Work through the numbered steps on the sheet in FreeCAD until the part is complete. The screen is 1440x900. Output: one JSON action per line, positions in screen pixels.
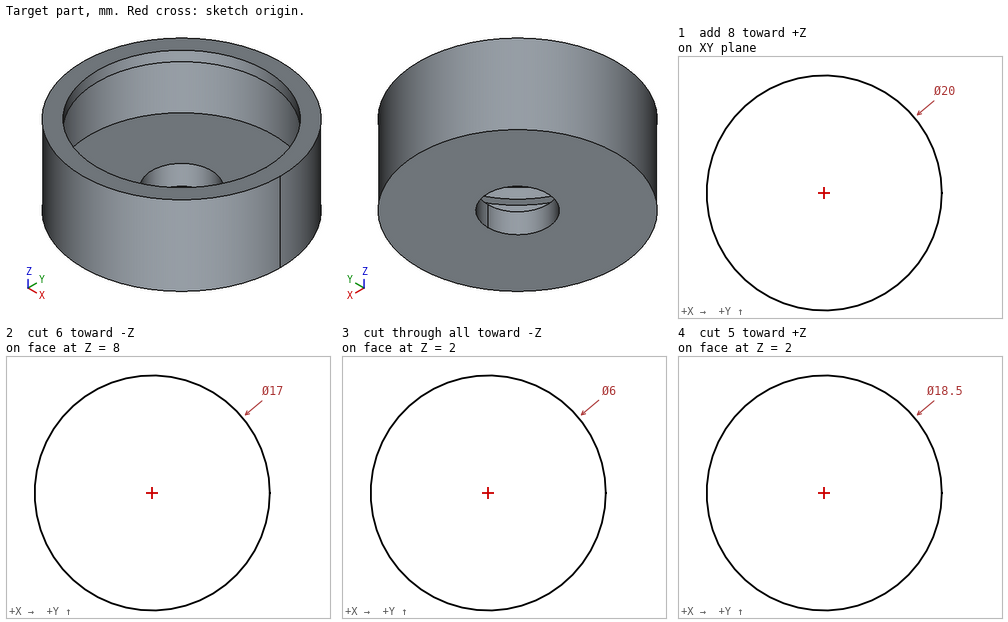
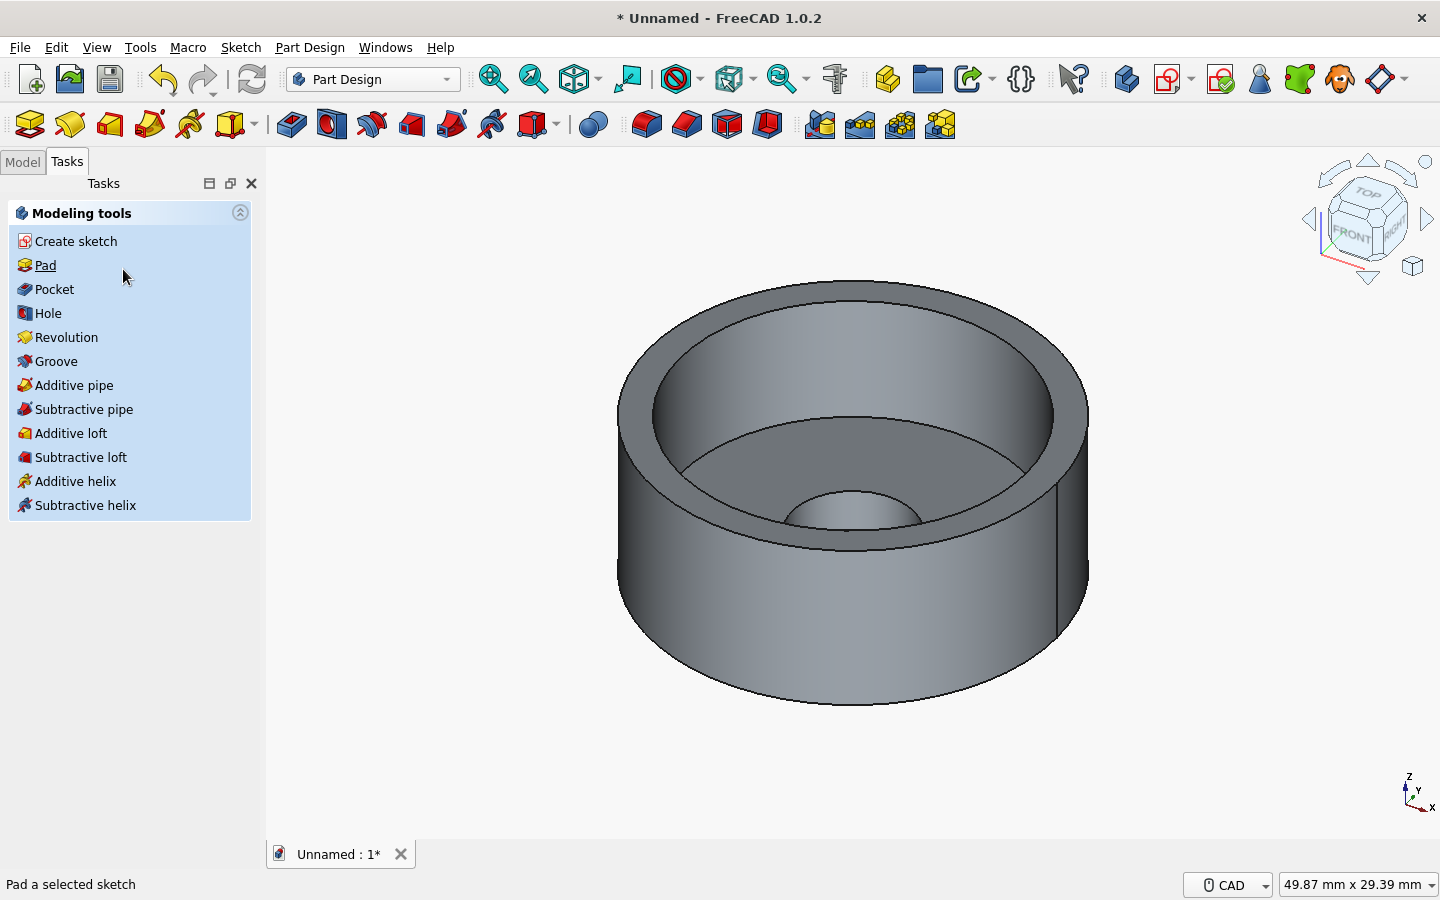
{"action": "left_click", "coordinate": [292, 124]}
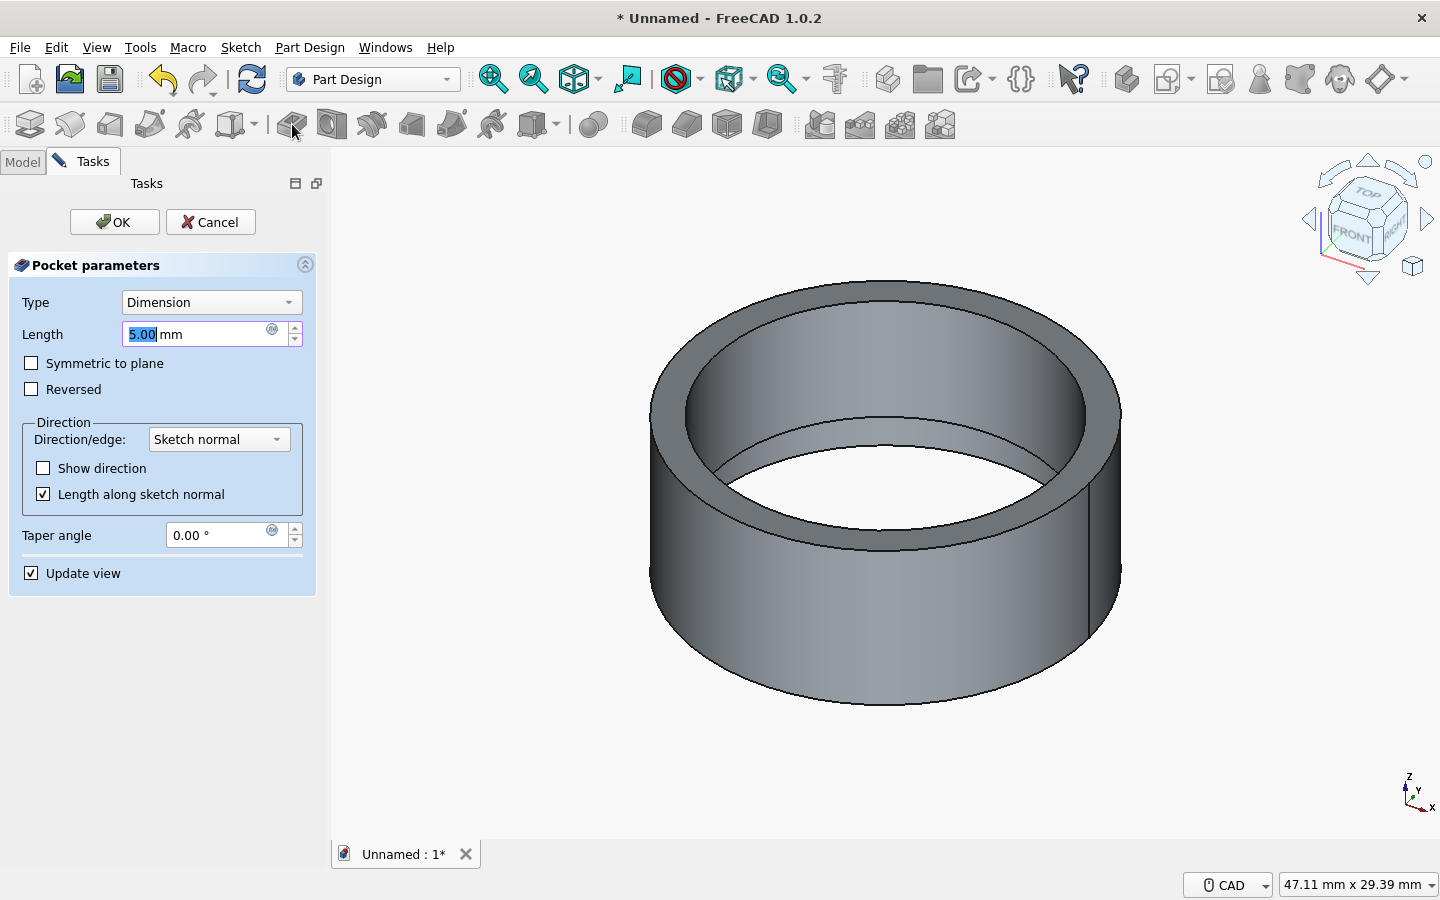
{"action": "type", "text": "5"}
{"action": "key", "text": "Tab"}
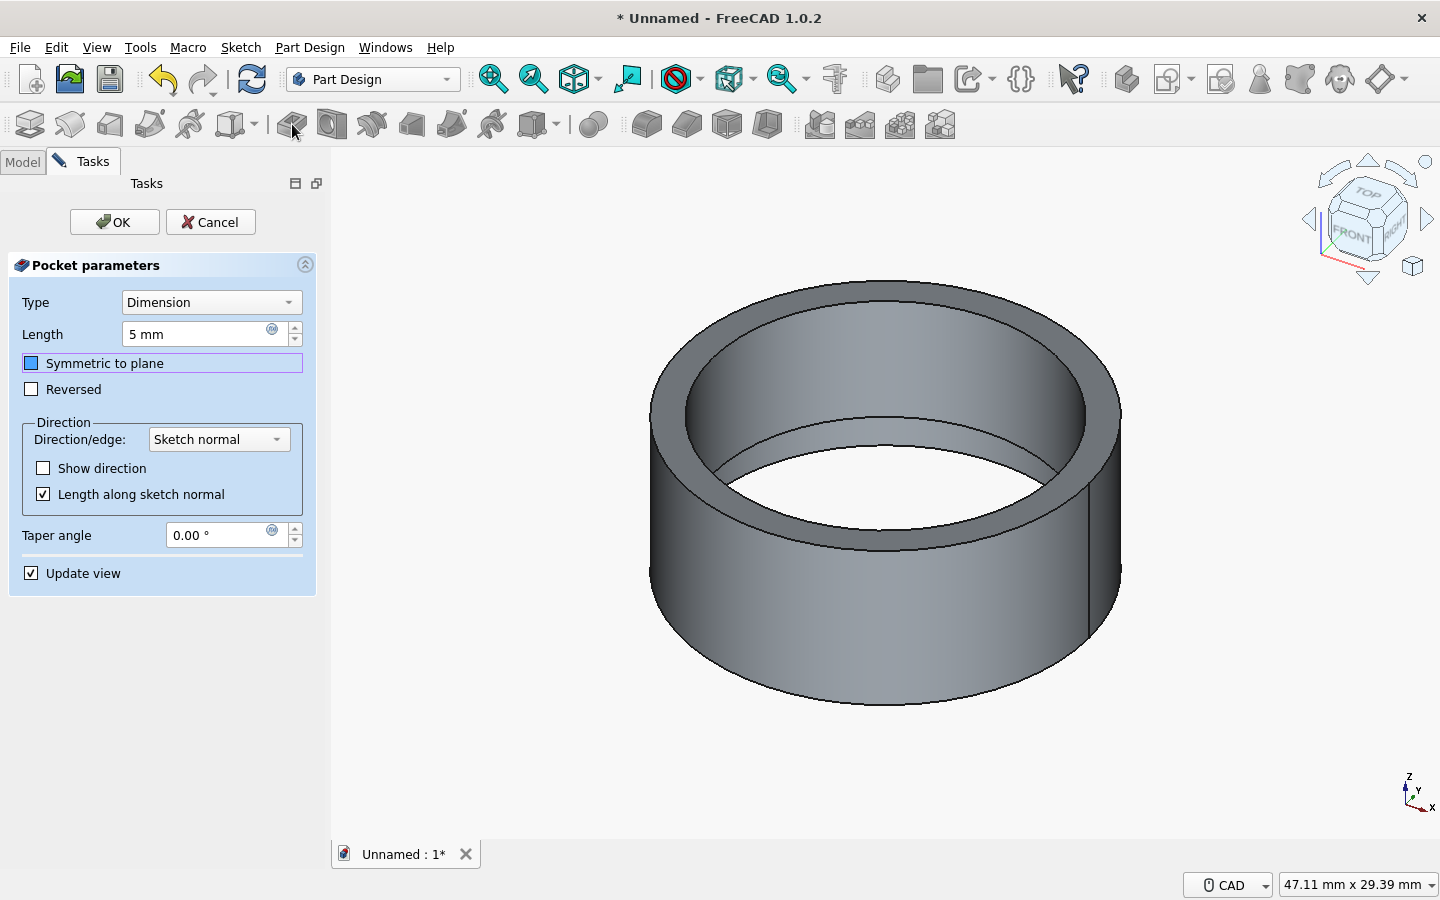
{"action": "left_click", "coordinate": [30, 389]}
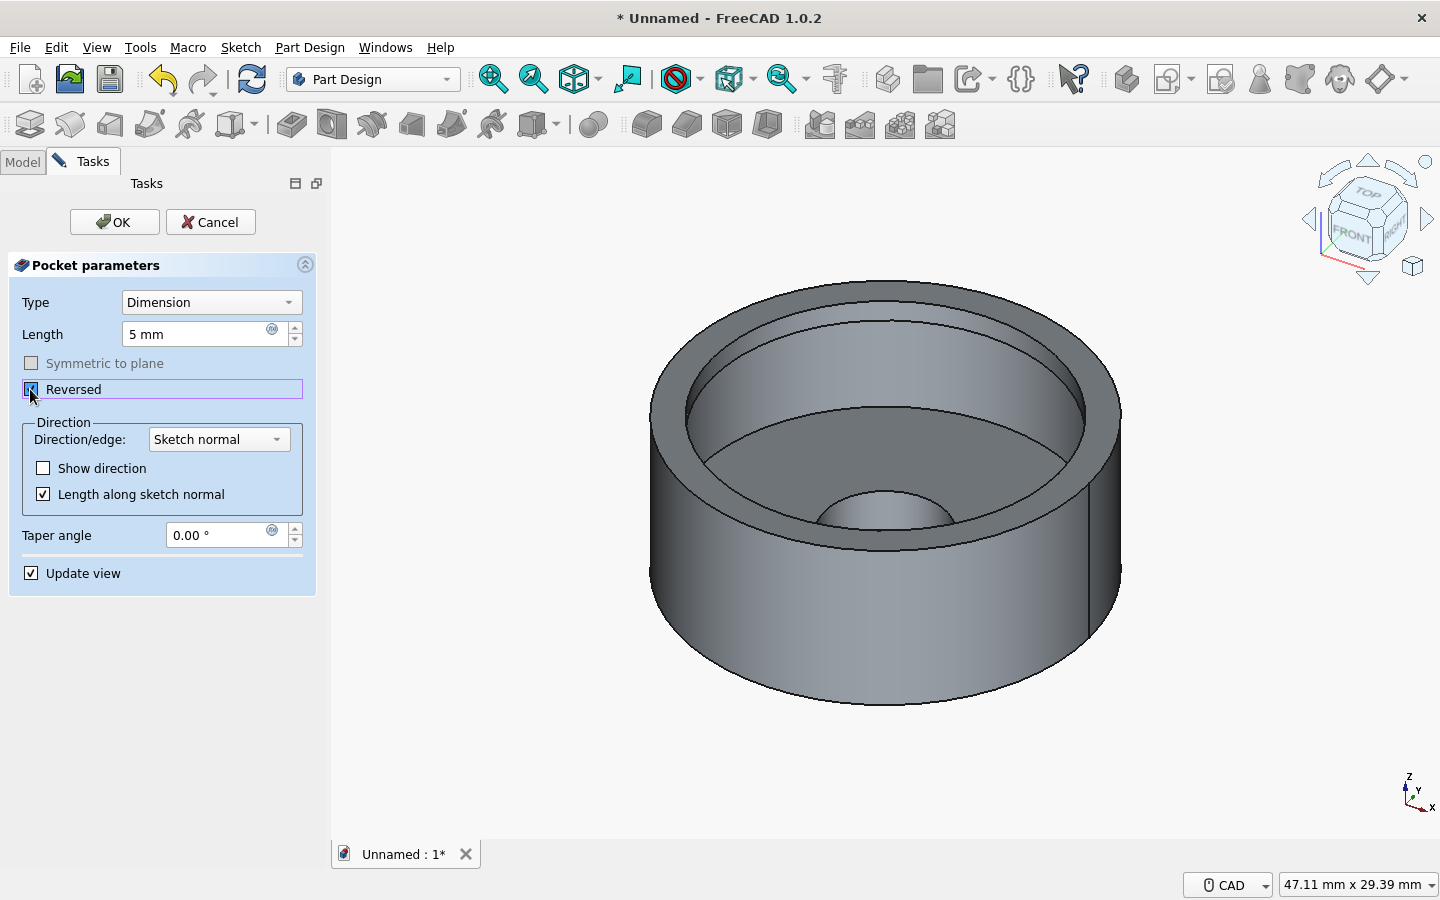
{"action": "left_click", "coordinate": [115, 222]}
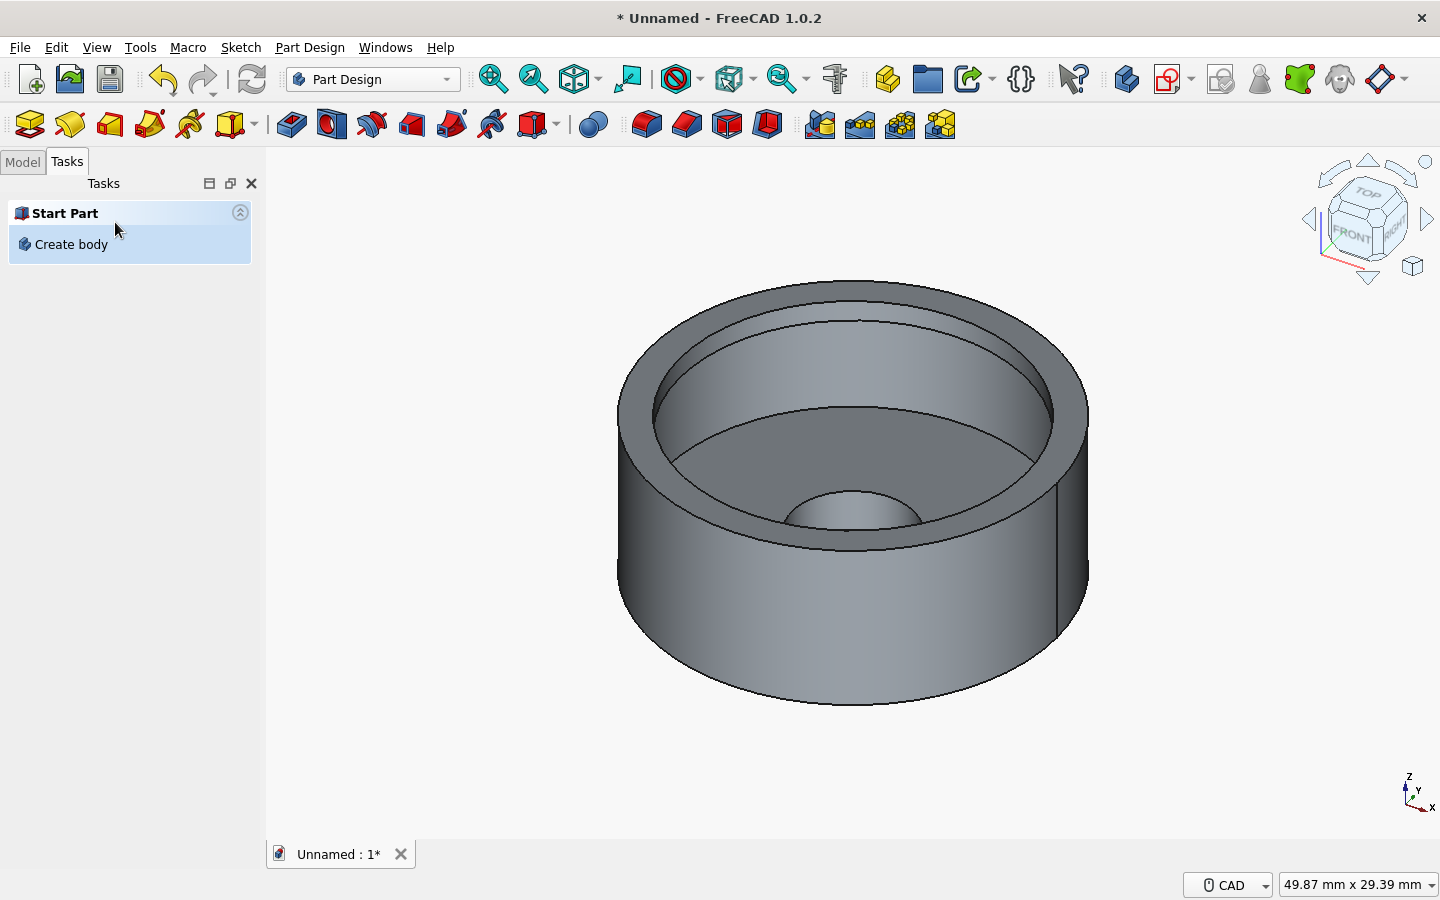
{"action": "key", "text": "0"}